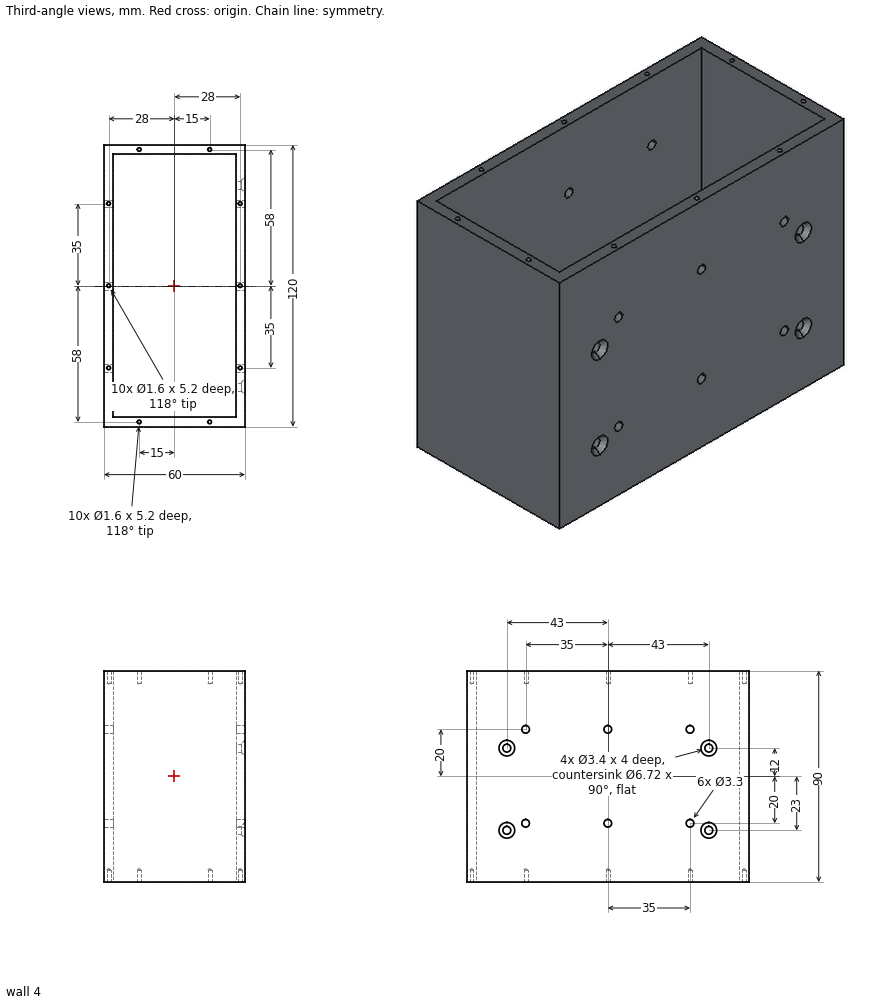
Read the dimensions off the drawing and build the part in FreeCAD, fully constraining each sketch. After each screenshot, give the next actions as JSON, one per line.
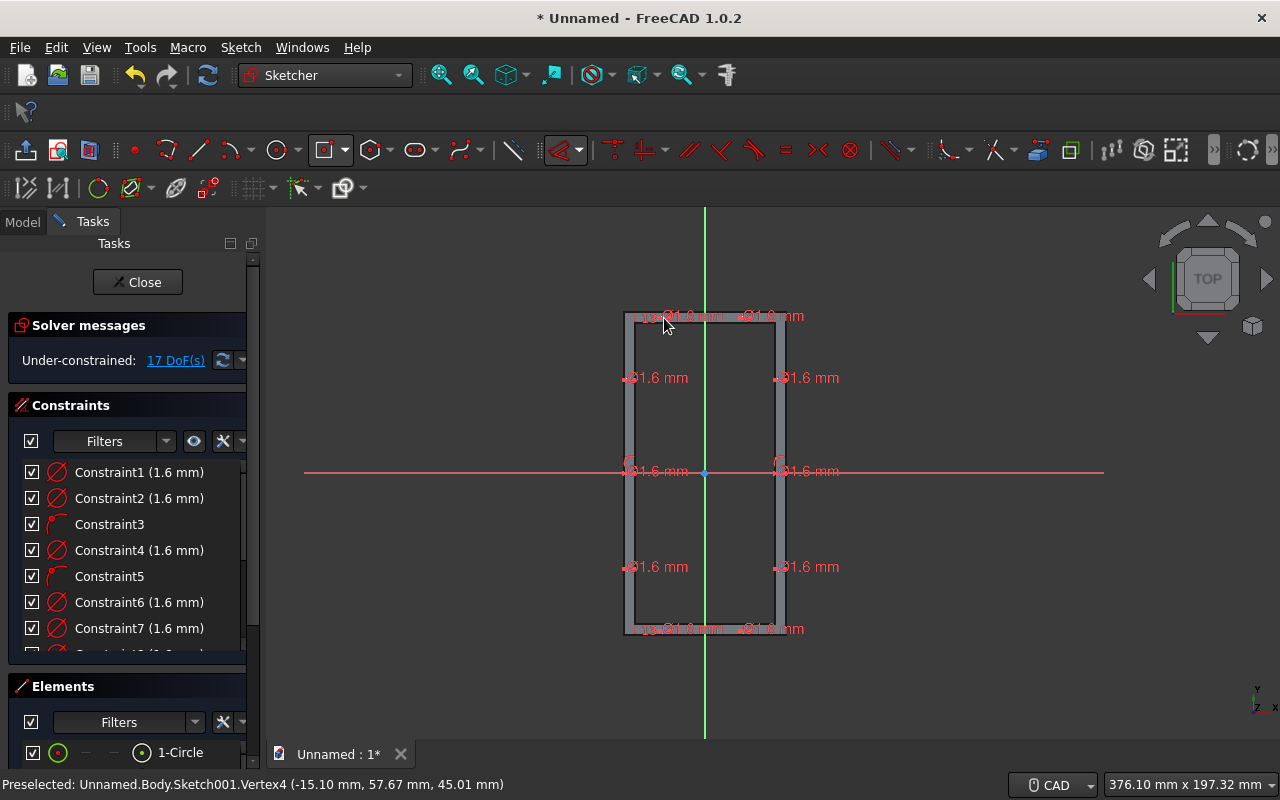
{"action": "left_click", "coordinate": [664, 318]}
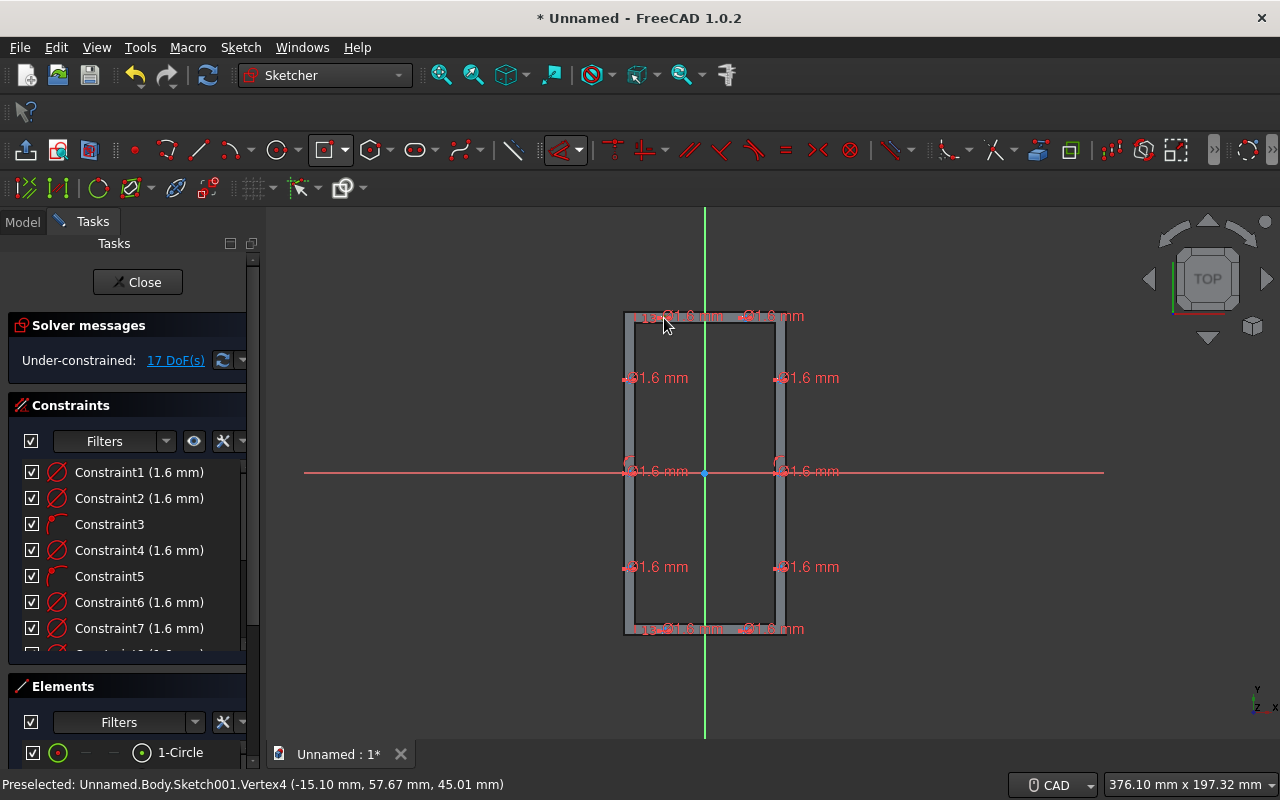
{"action": "left_click", "coordinate": [745, 318]}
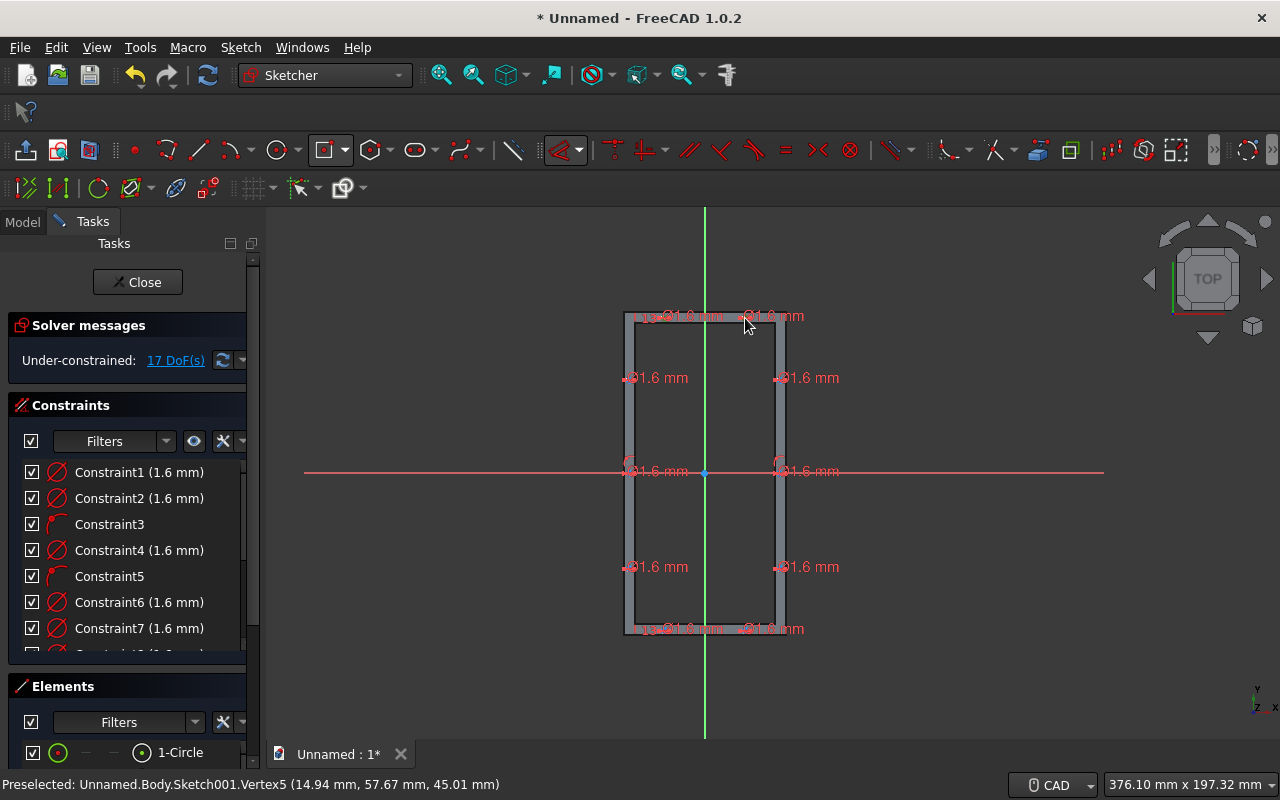
{"action": "left_click", "coordinate": [668, 150]}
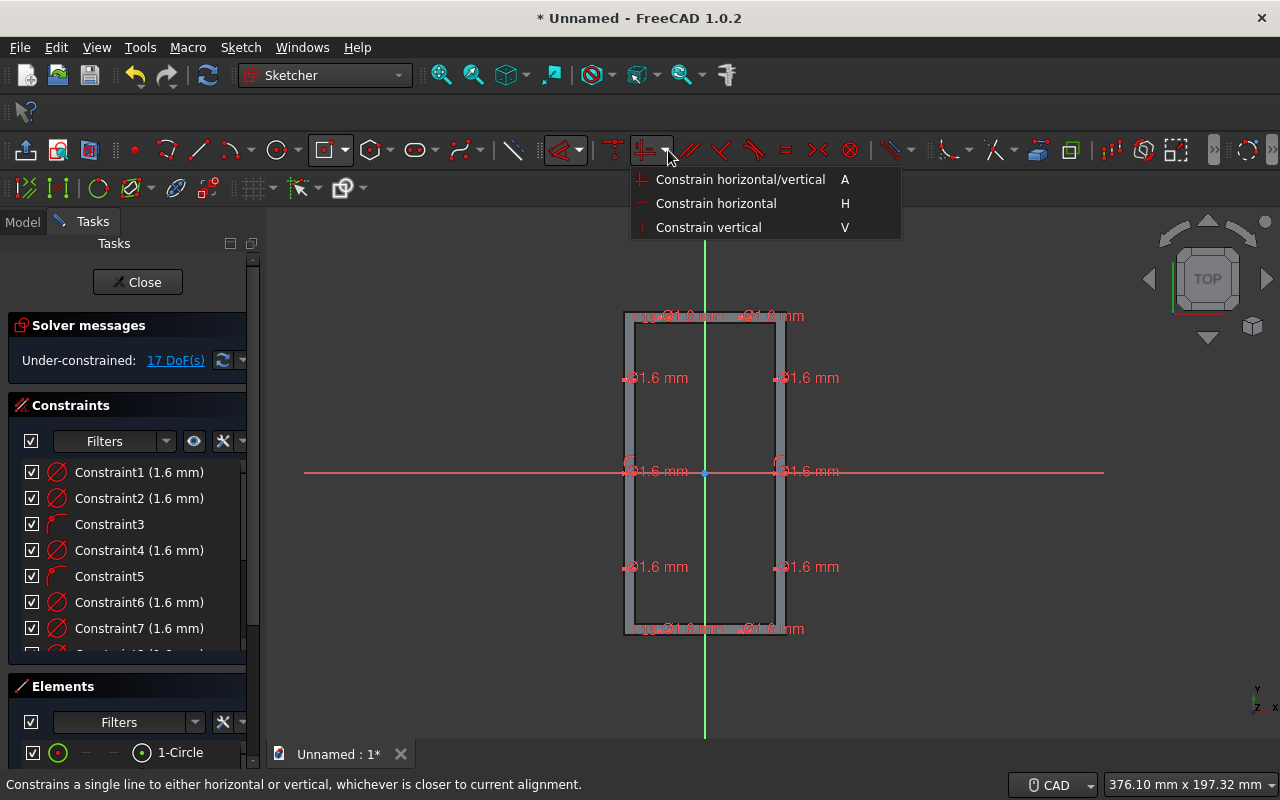
{"action": "left_click", "coordinate": [766, 203]}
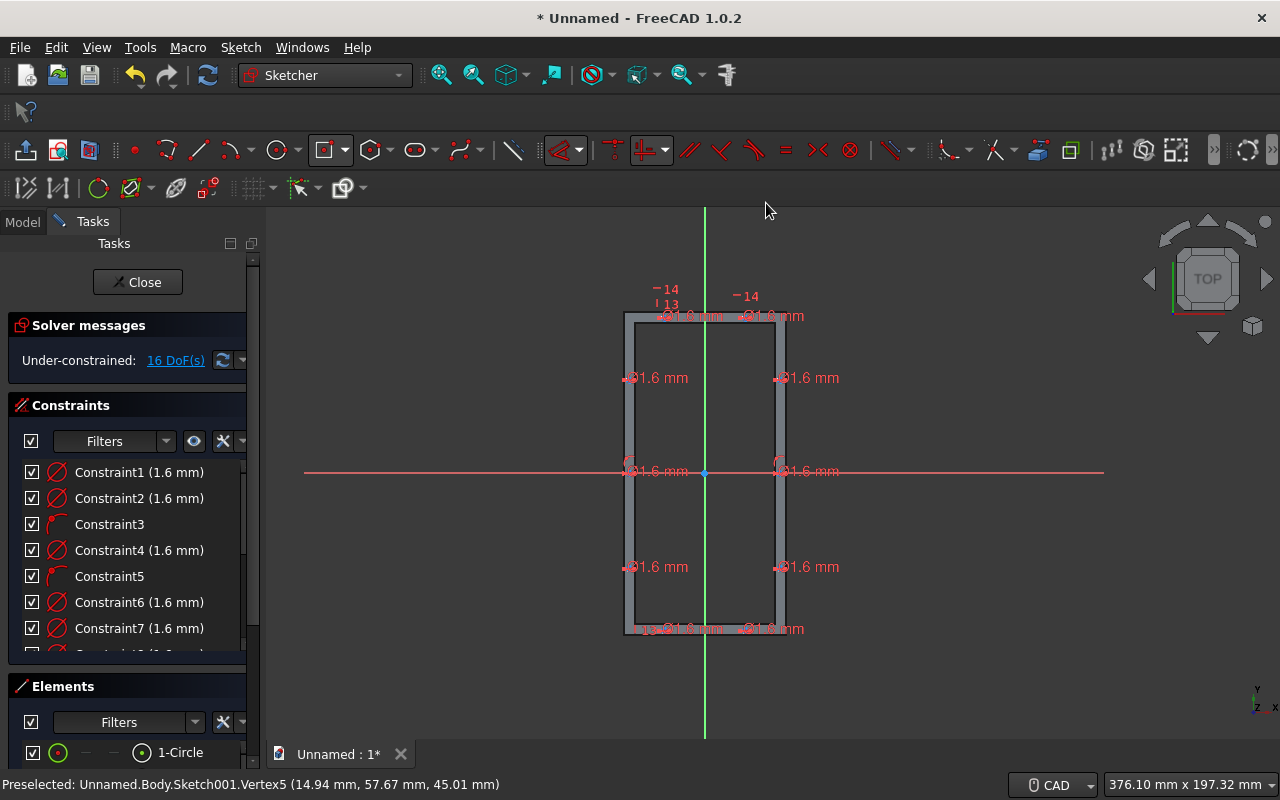
{"action": "left_click", "coordinate": [629, 473]}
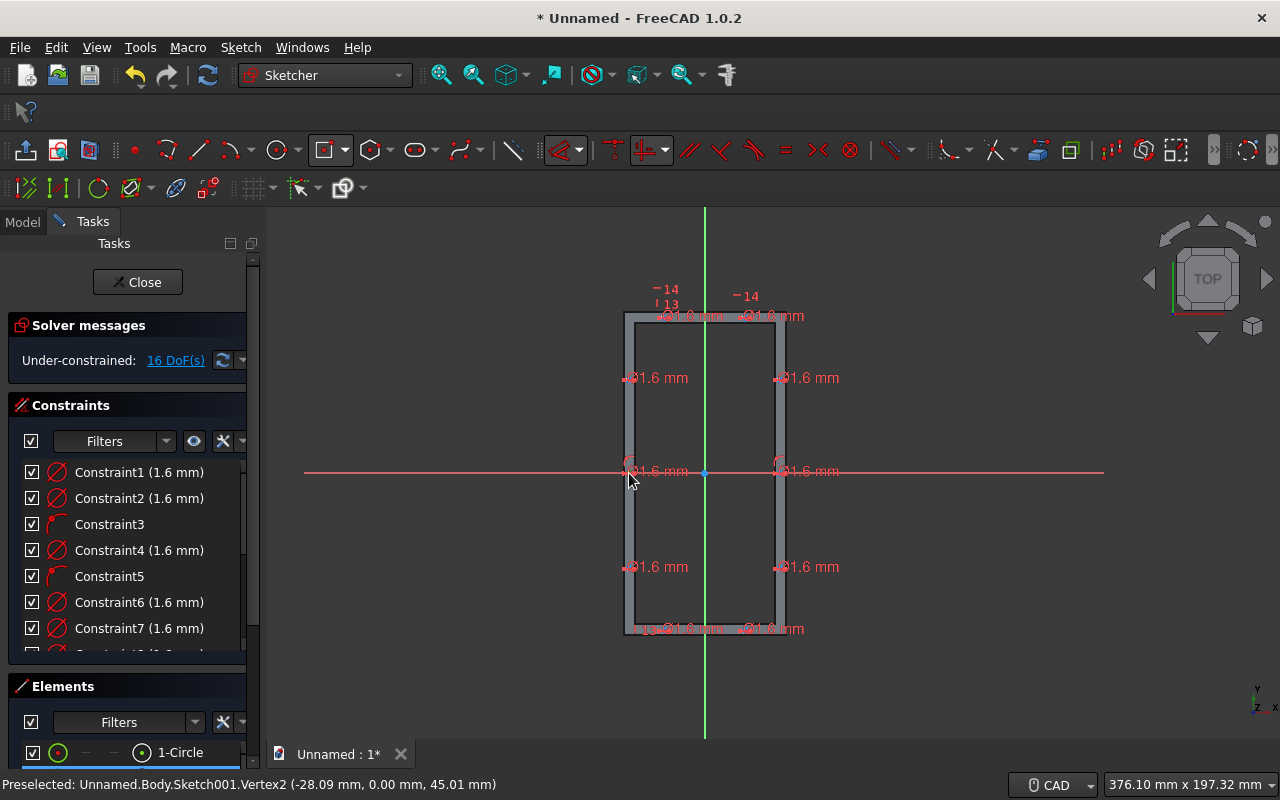
{"action": "left_click", "coordinate": [629, 380]}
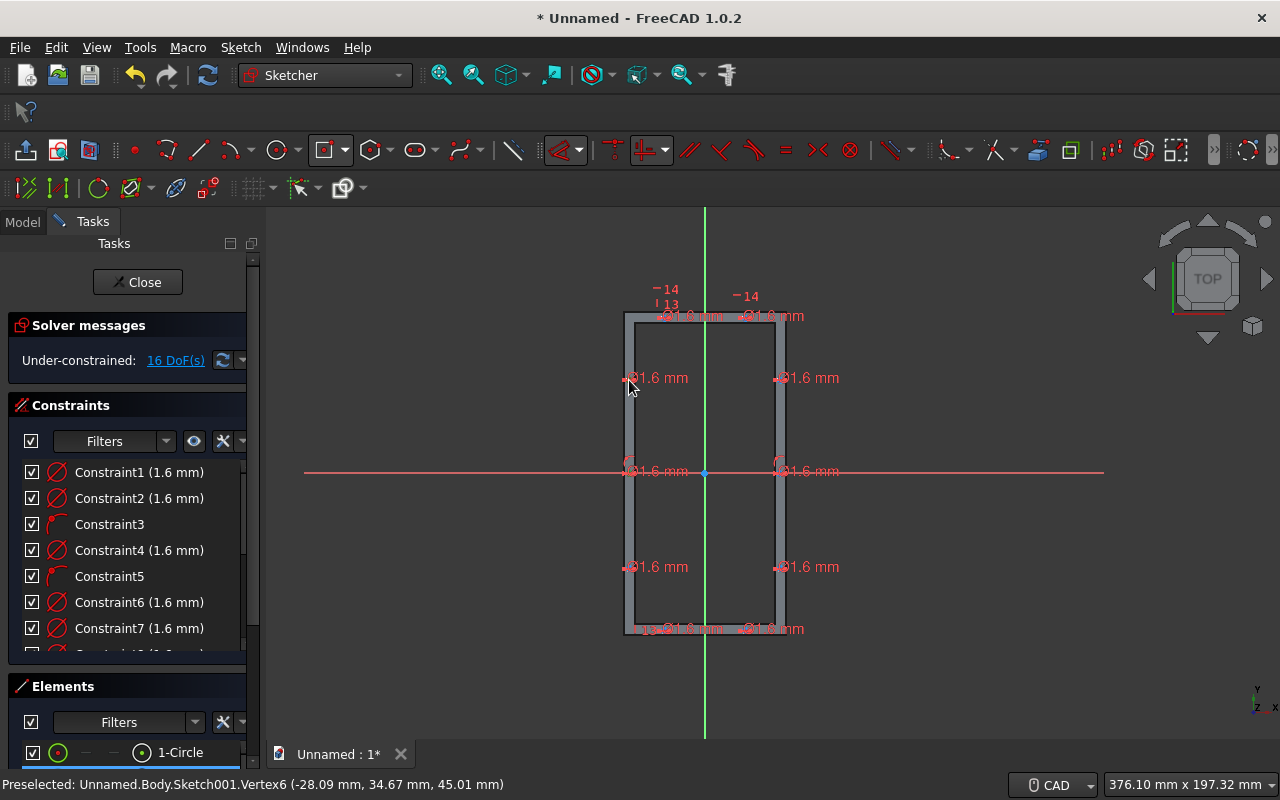
{"action": "left_click", "coordinate": [668, 150]}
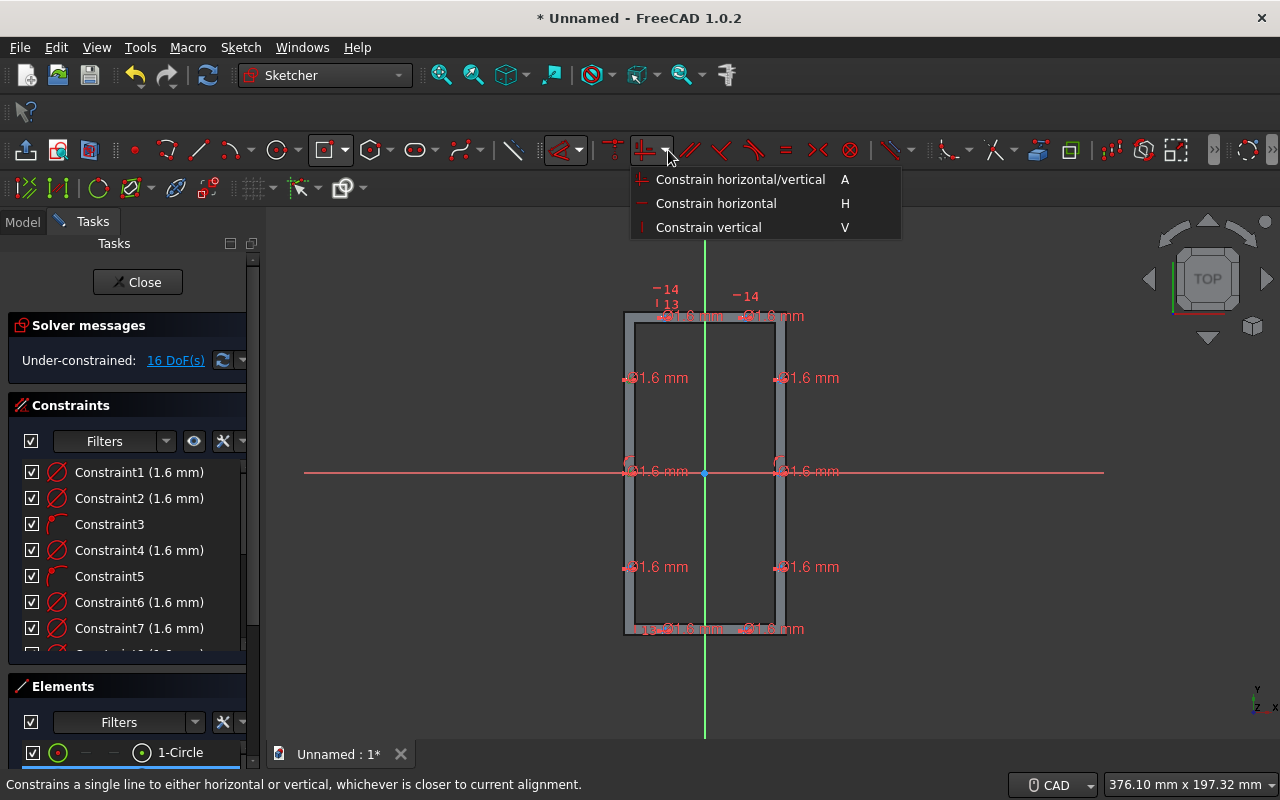
{"action": "left_click", "coordinate": [766, 227]}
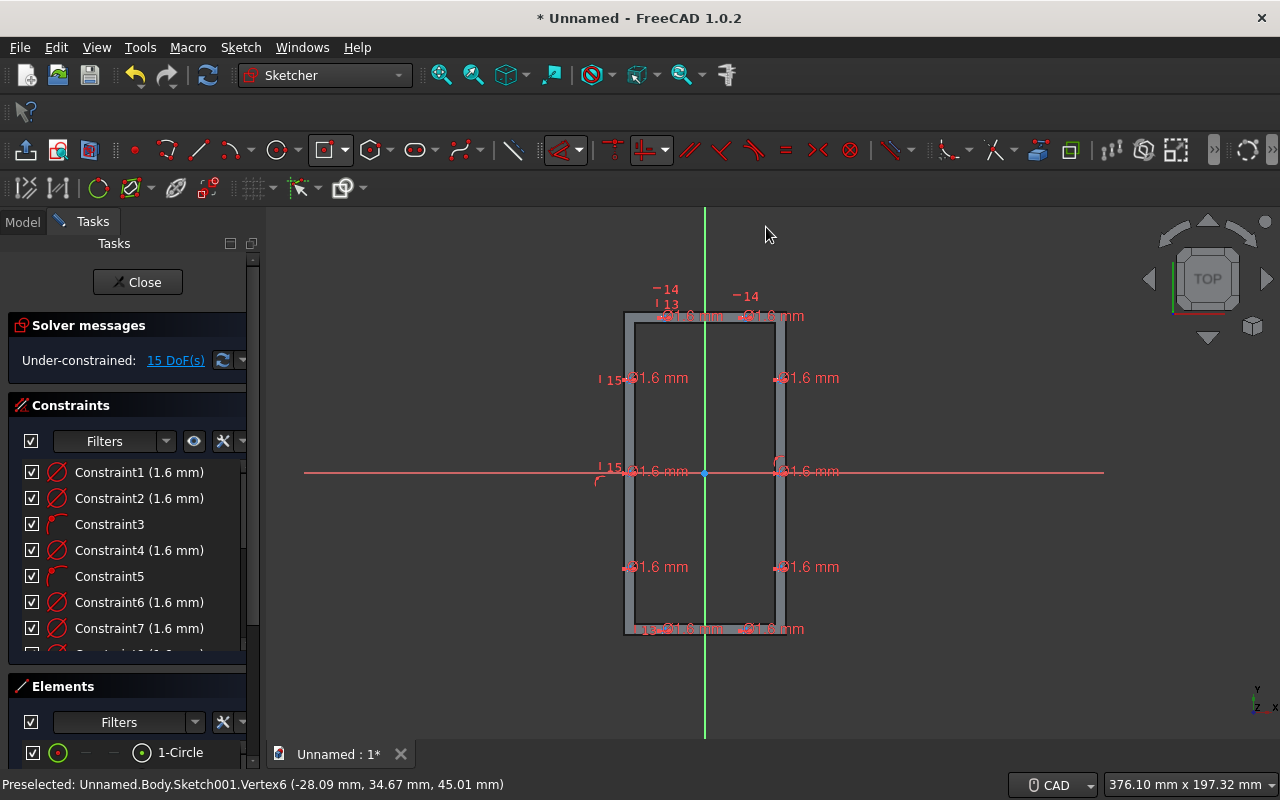
{"action": "left_click", "coordinate": [780, 473]}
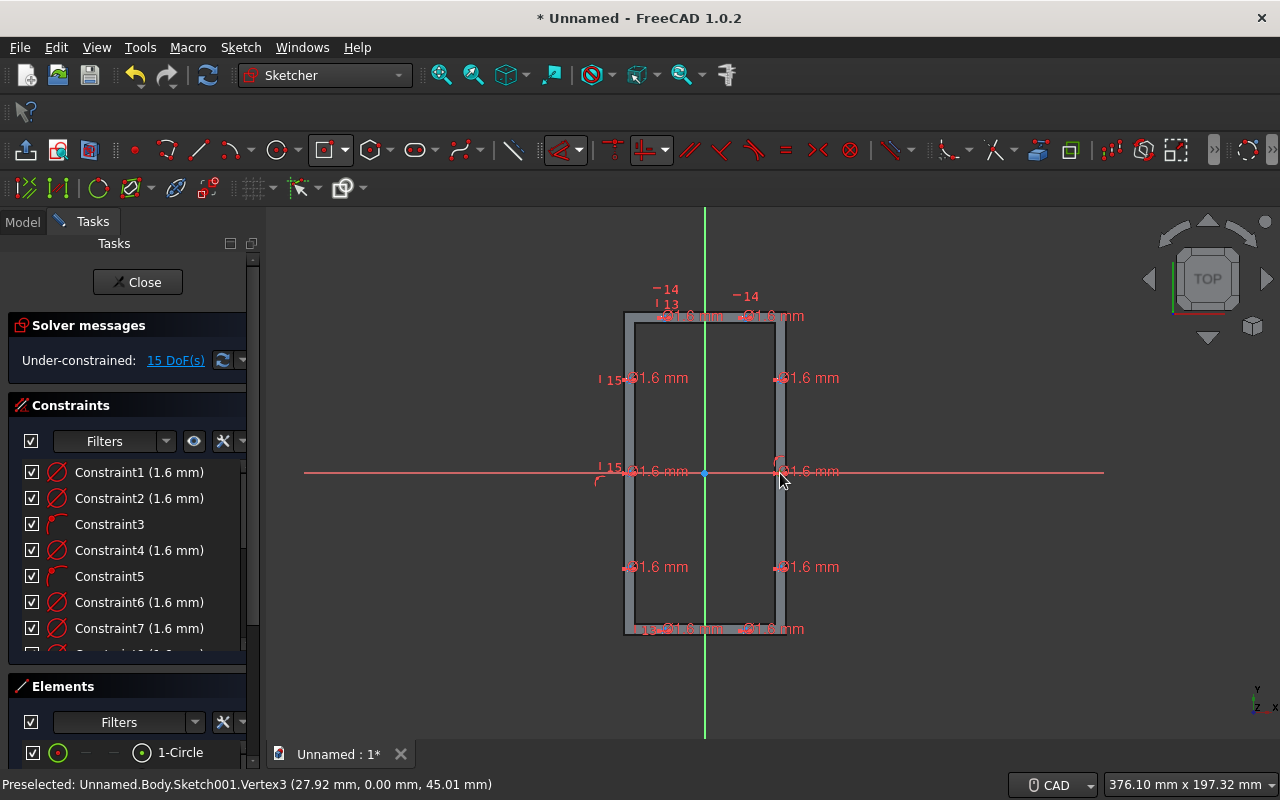
{"action": "left_click", "coordinate": [780, 380]}